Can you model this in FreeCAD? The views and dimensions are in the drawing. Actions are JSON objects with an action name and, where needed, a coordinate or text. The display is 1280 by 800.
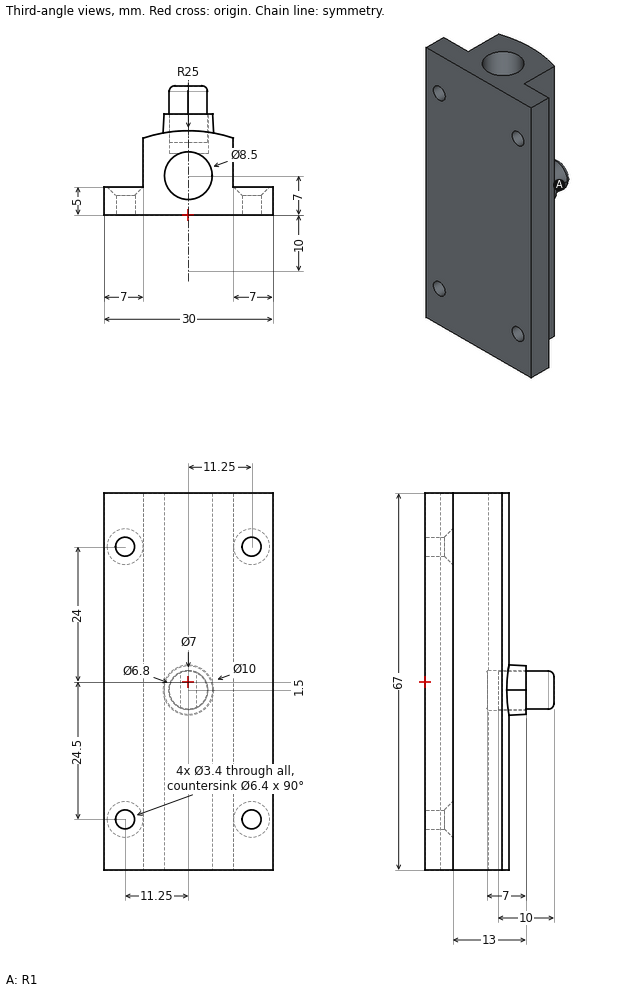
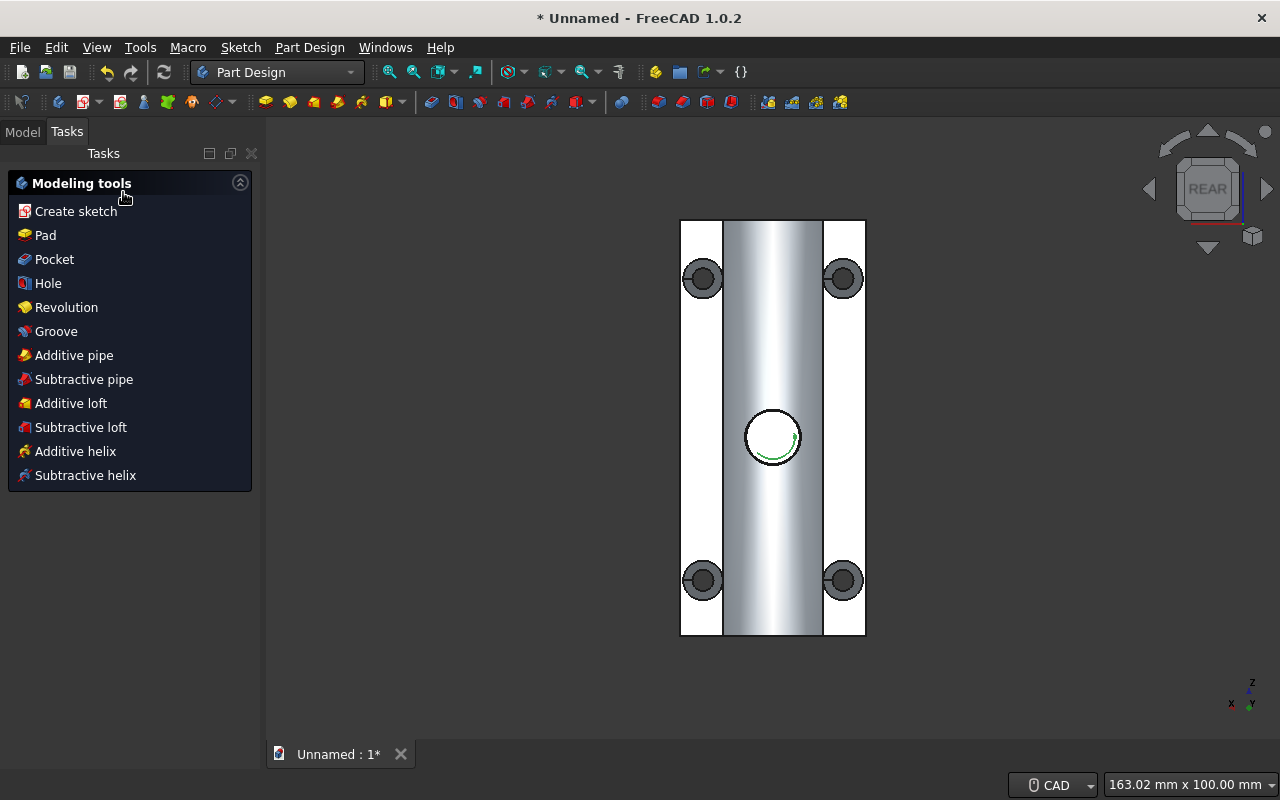
{"action": "left_click", "coordinate": [432, 102]}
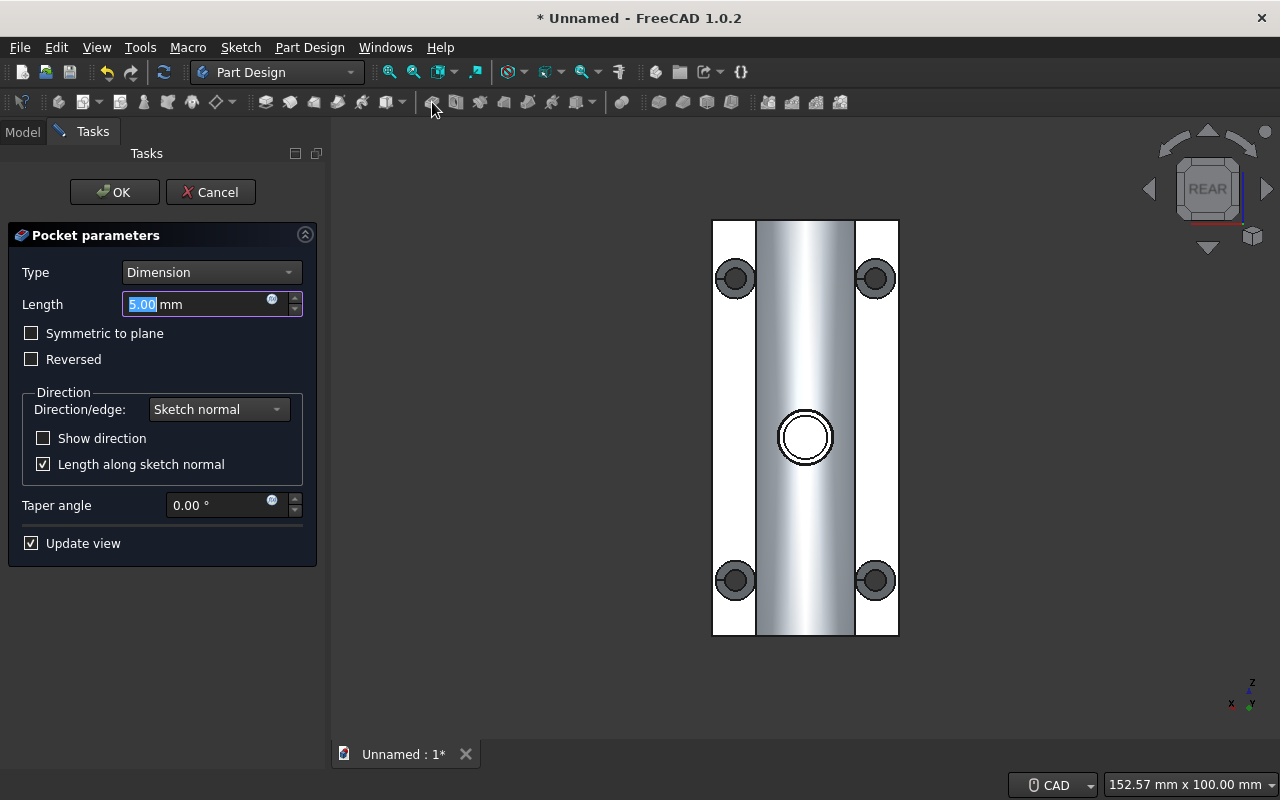
{"action": "type", "text": "7"}
{"action": "key", "text": "Tab"}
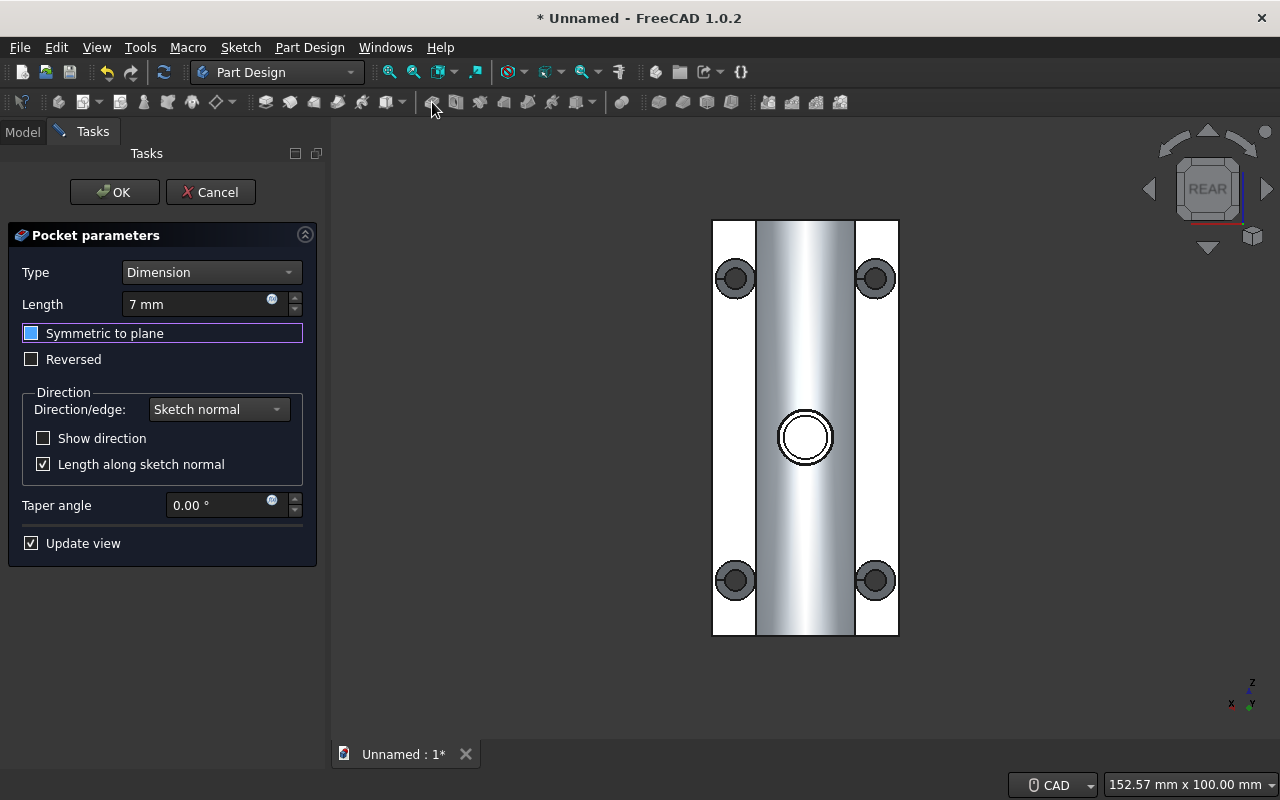
{"action": "left_click", "coordinate": [115, 192]}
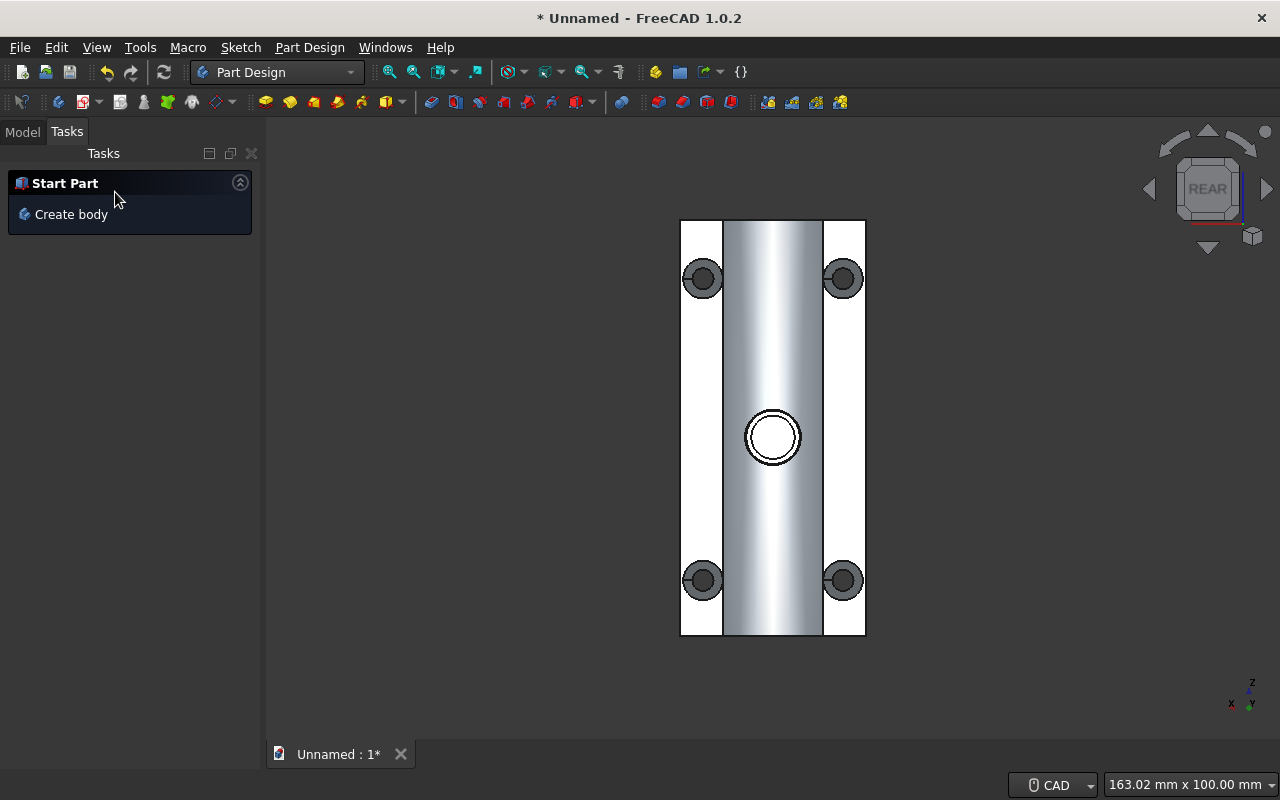
{"action": "key", "text": "0"}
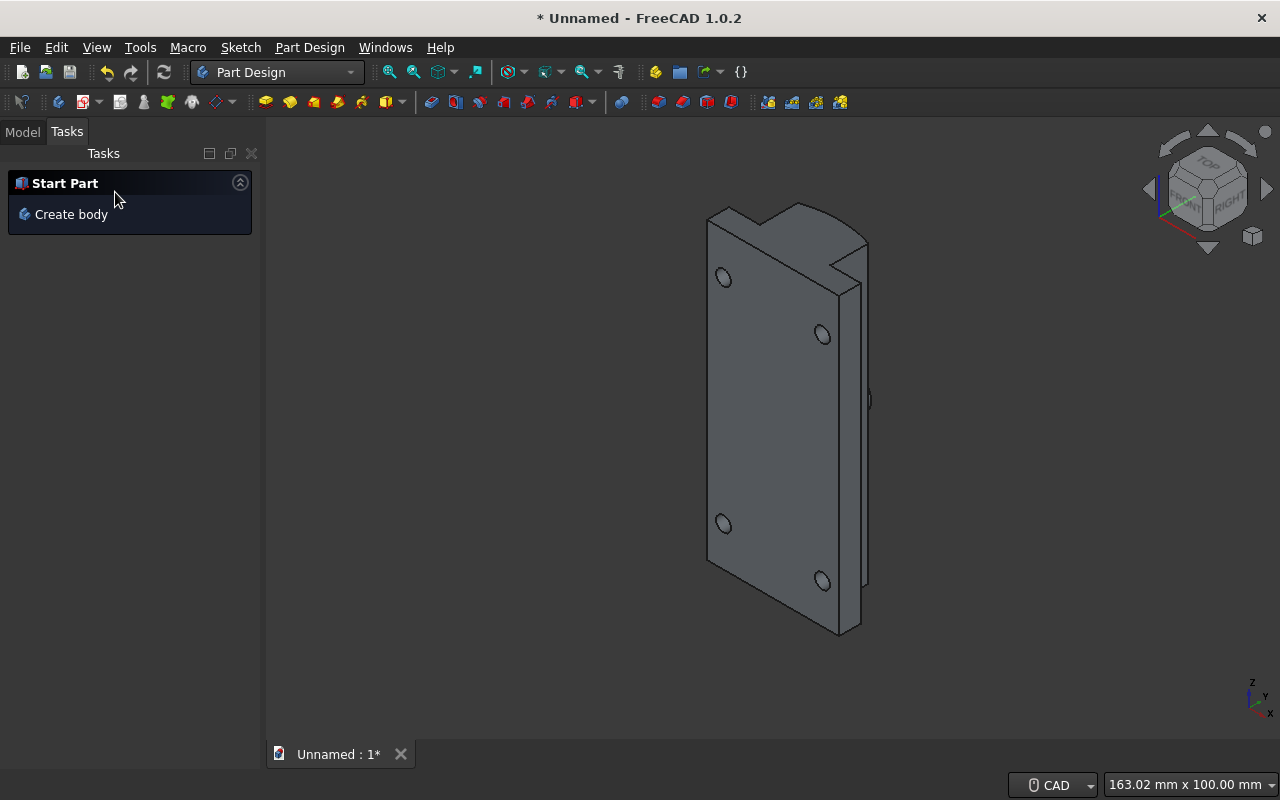
{"action": "left_click", "coordinate": [806, 238]}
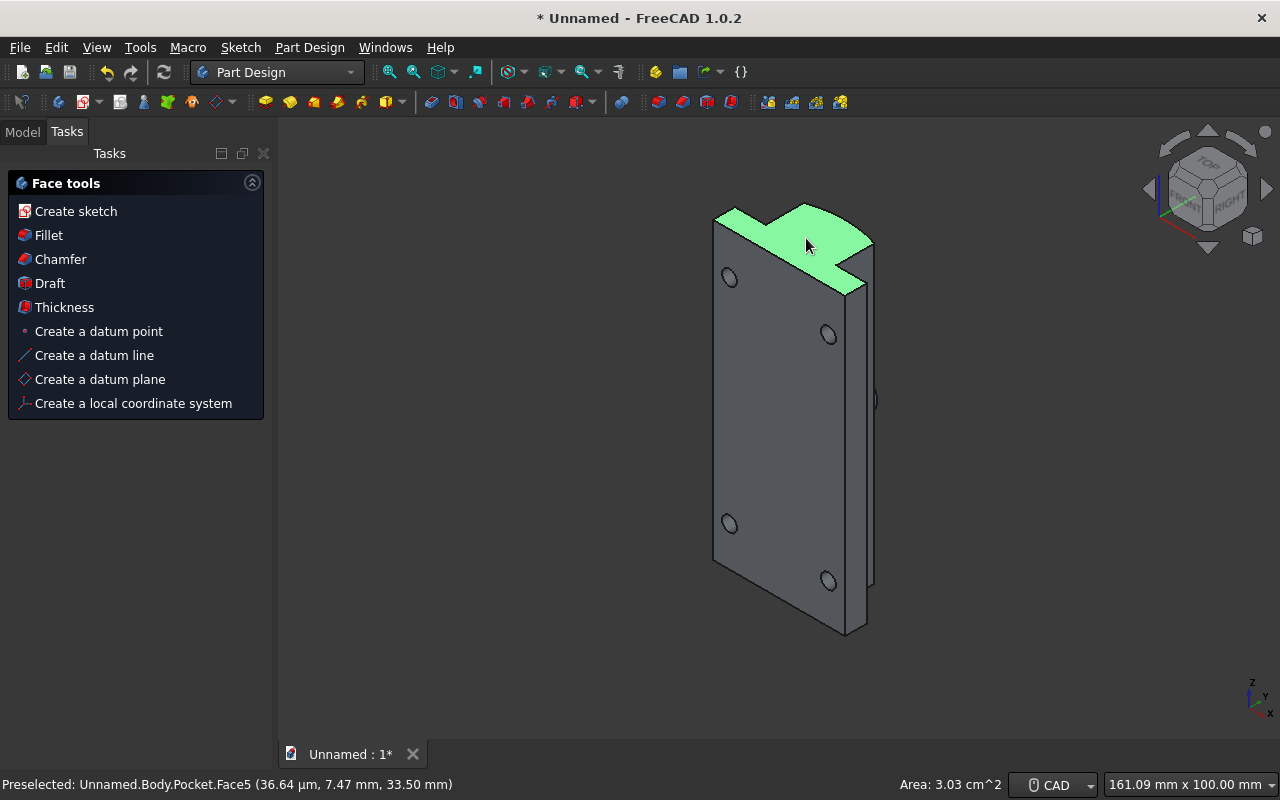
{"action": "left_click", "coordinate": [84, 102]}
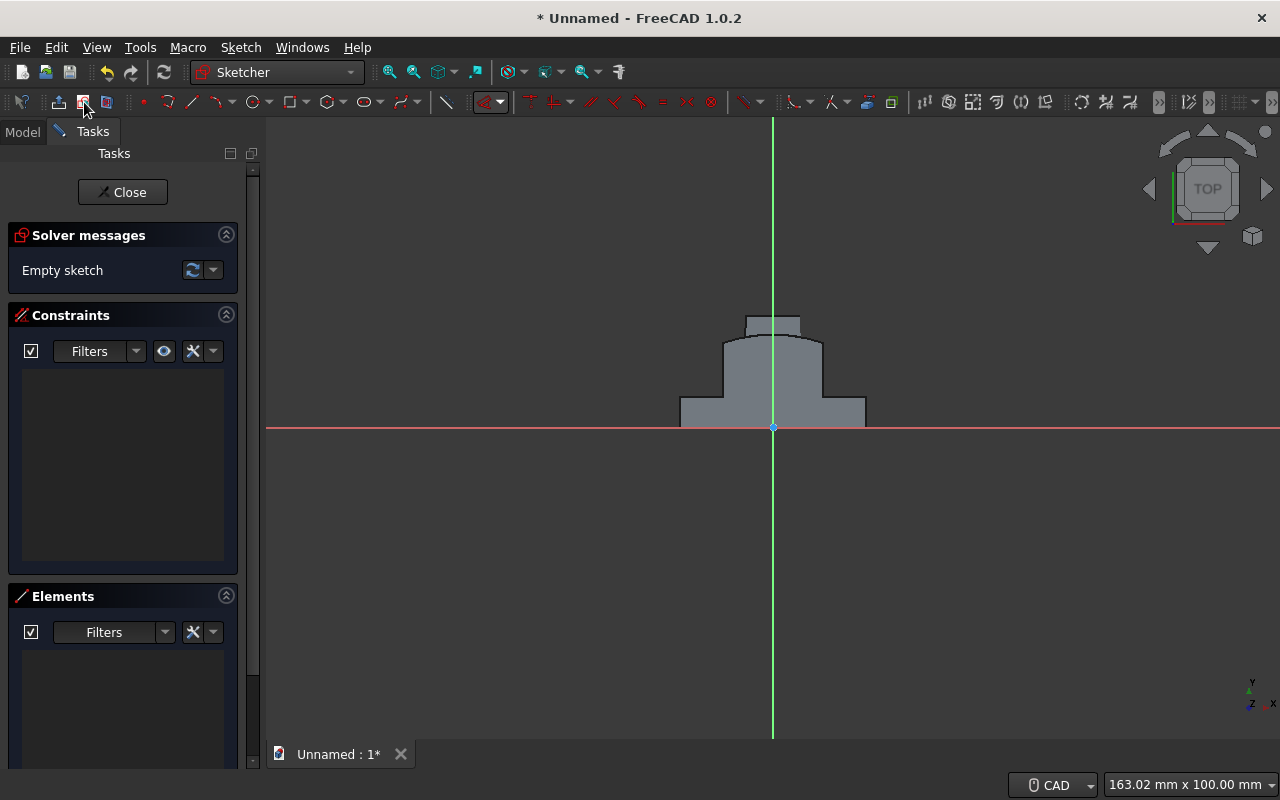
{"action": "scroll", "coordinate": [787, 386], "scroll_direction": "up", "scroll_amount": 9}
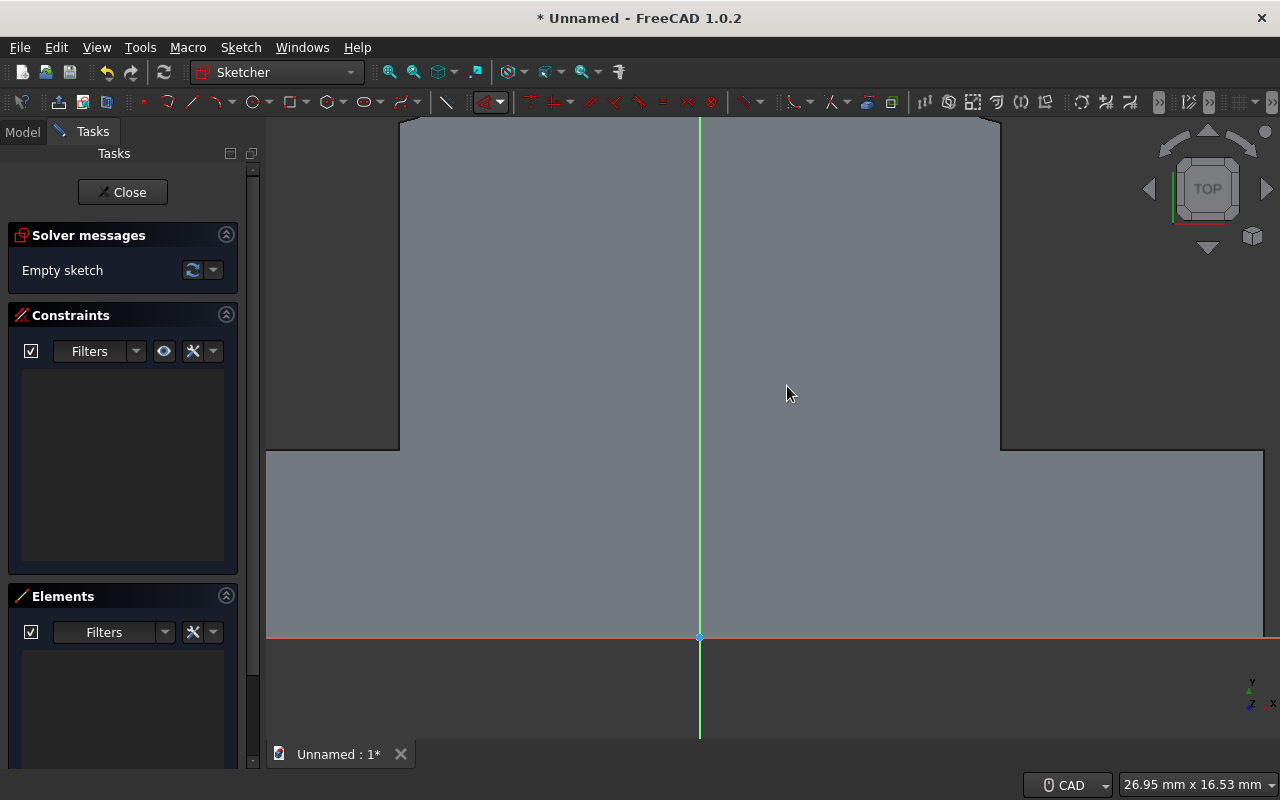
{"action": "left_click", "coordinate": [254, 102]}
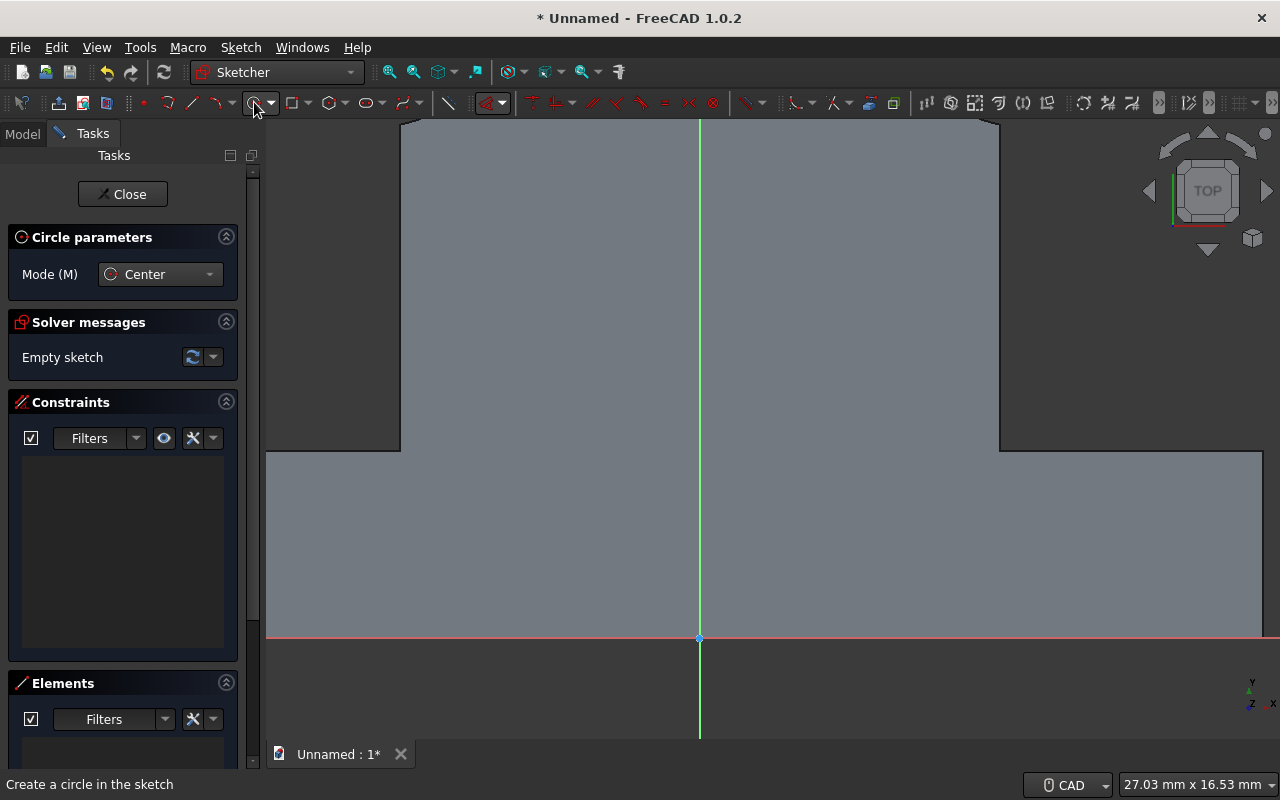
{"action": "left_click", "coordinate": [700, 376]}
{"action": "left_click", "coordinate": [813, 263]}
{"action": "key", "text": "Escape"}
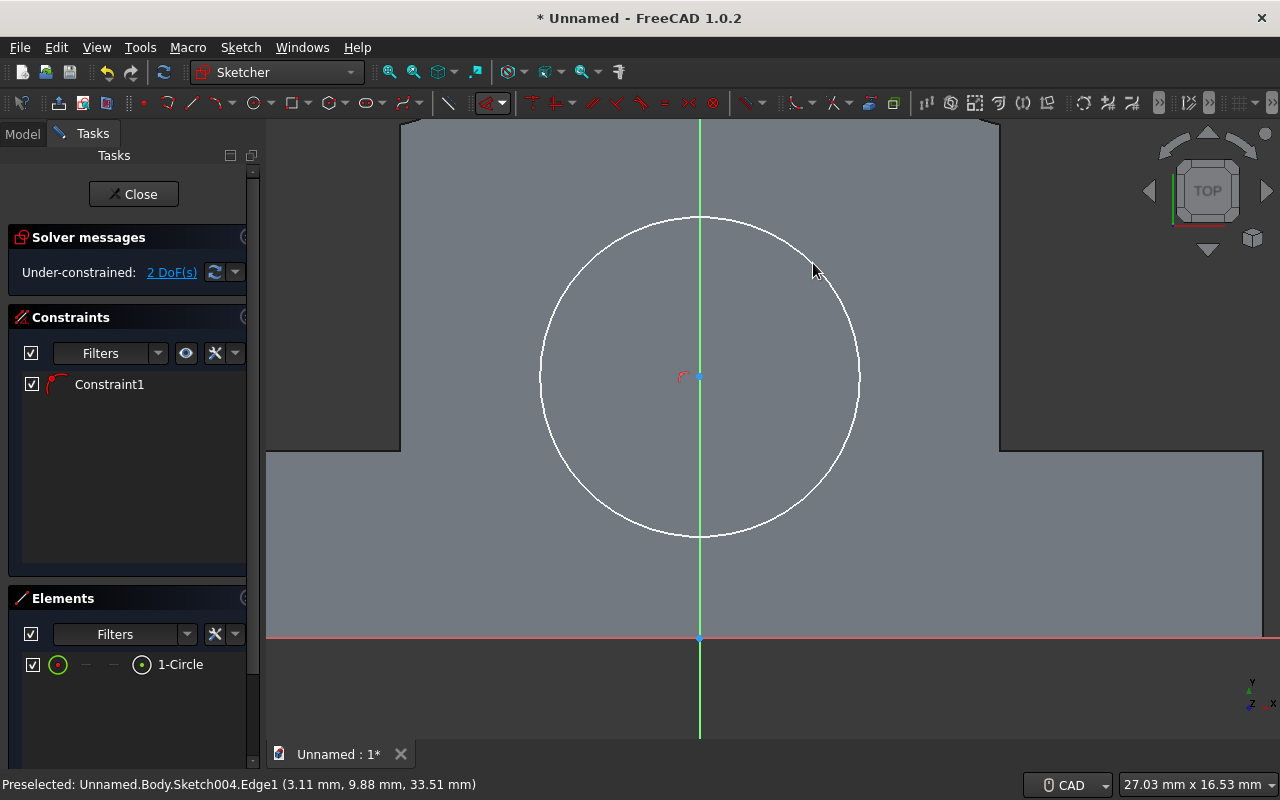
{"action": "left_click", "coordinate": [813, 264]}